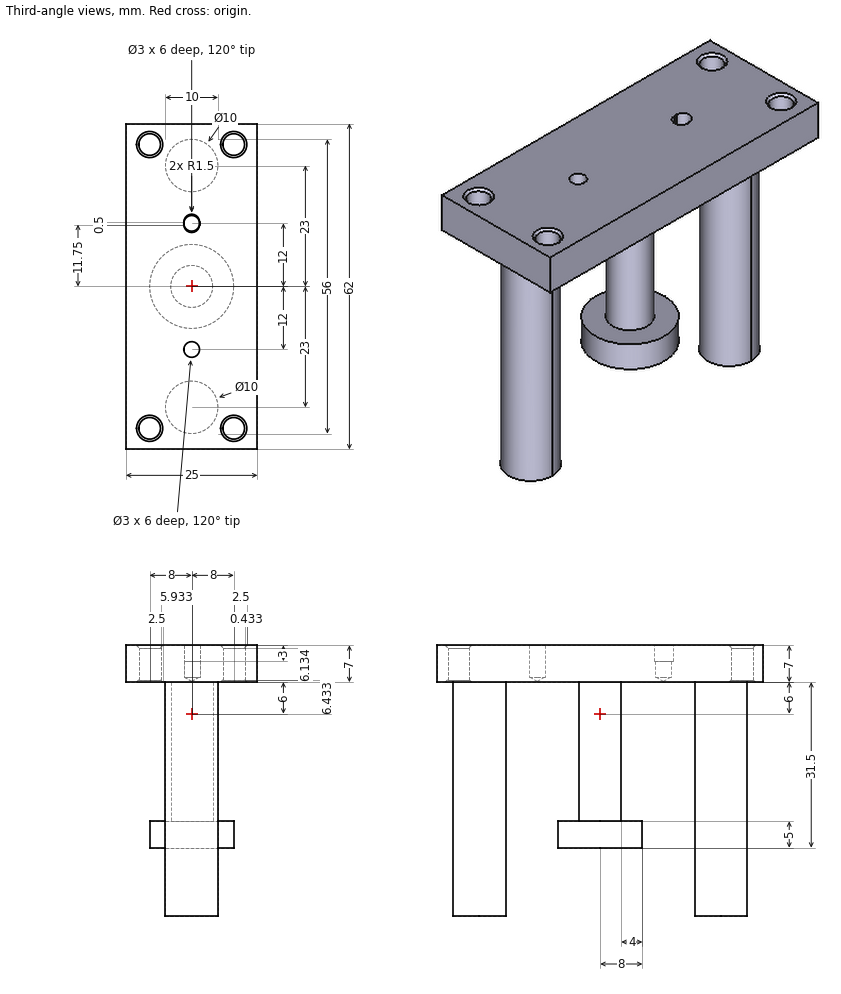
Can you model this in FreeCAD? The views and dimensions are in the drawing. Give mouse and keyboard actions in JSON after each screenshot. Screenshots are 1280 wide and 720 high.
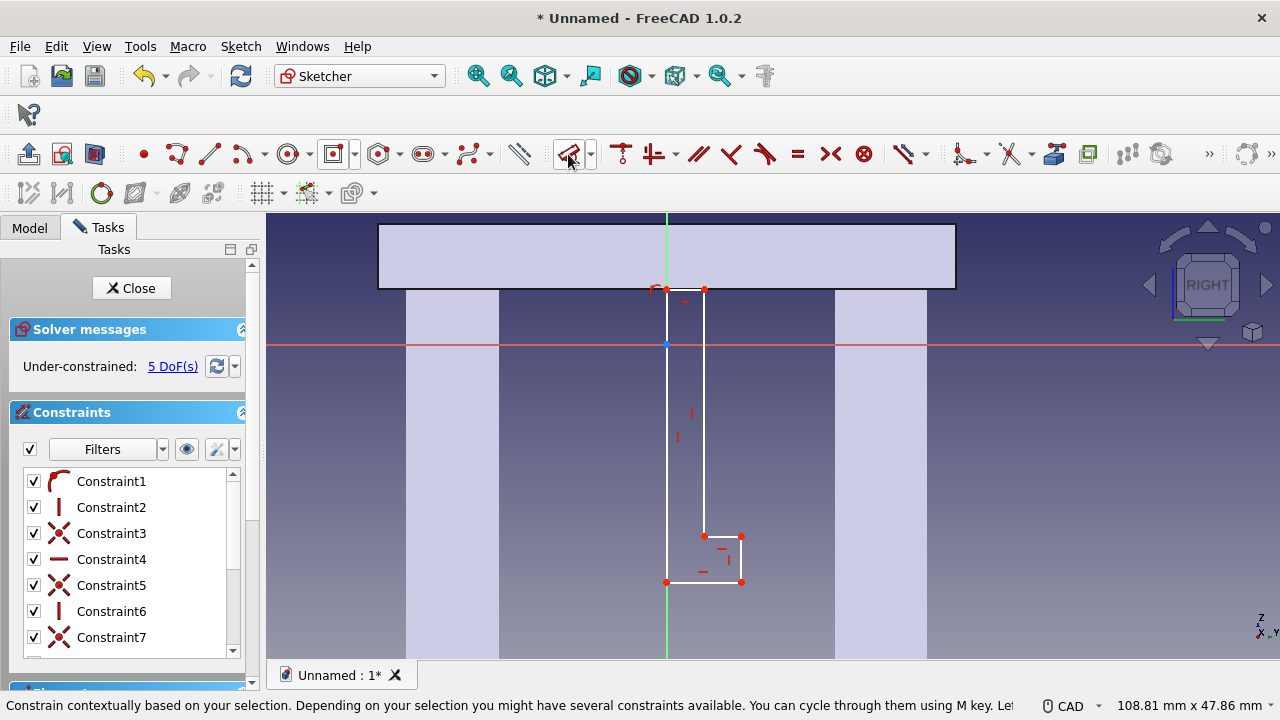
{"action": "left_click", "coordinate": [689, 583]}
{"action": "left_click", "coordinate": [704, 617]}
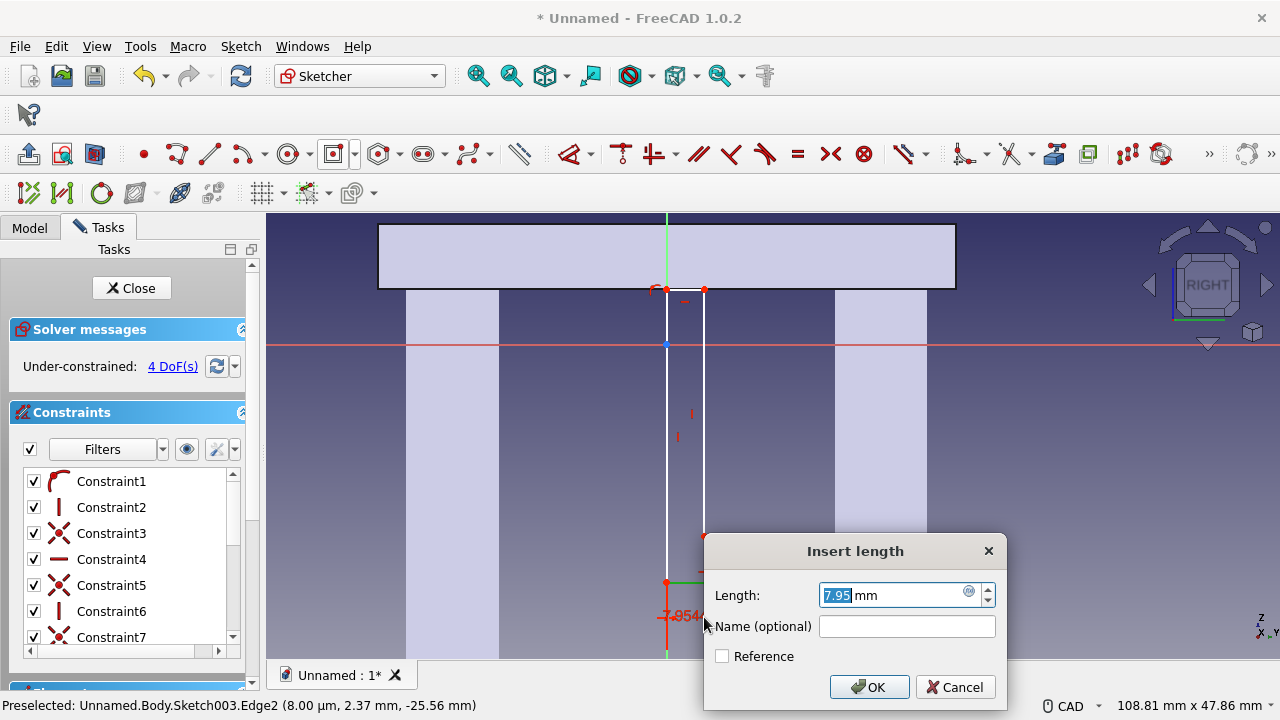
{"action": "type", "text": "8"}
{"action": "key", "text": "Return"}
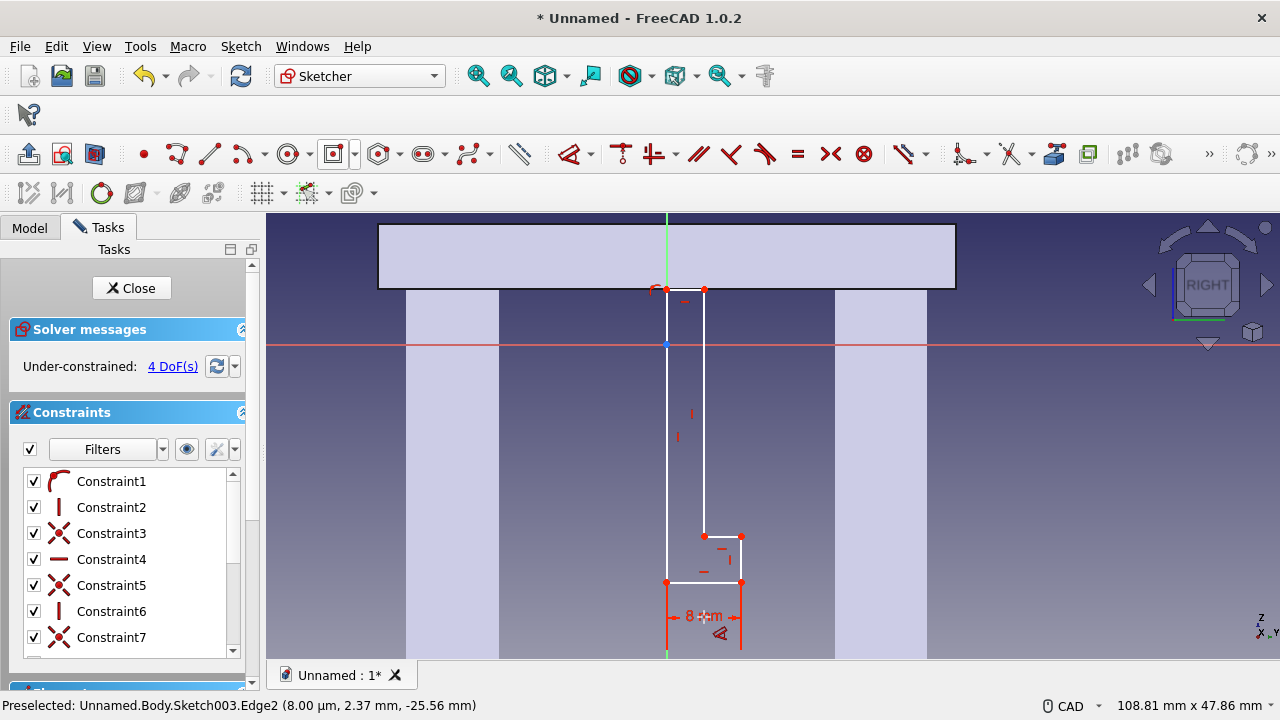
{"action": "left_click", "coordinate": [741, 569]}
{"action": "left_click", "coordinate": [775, 560]}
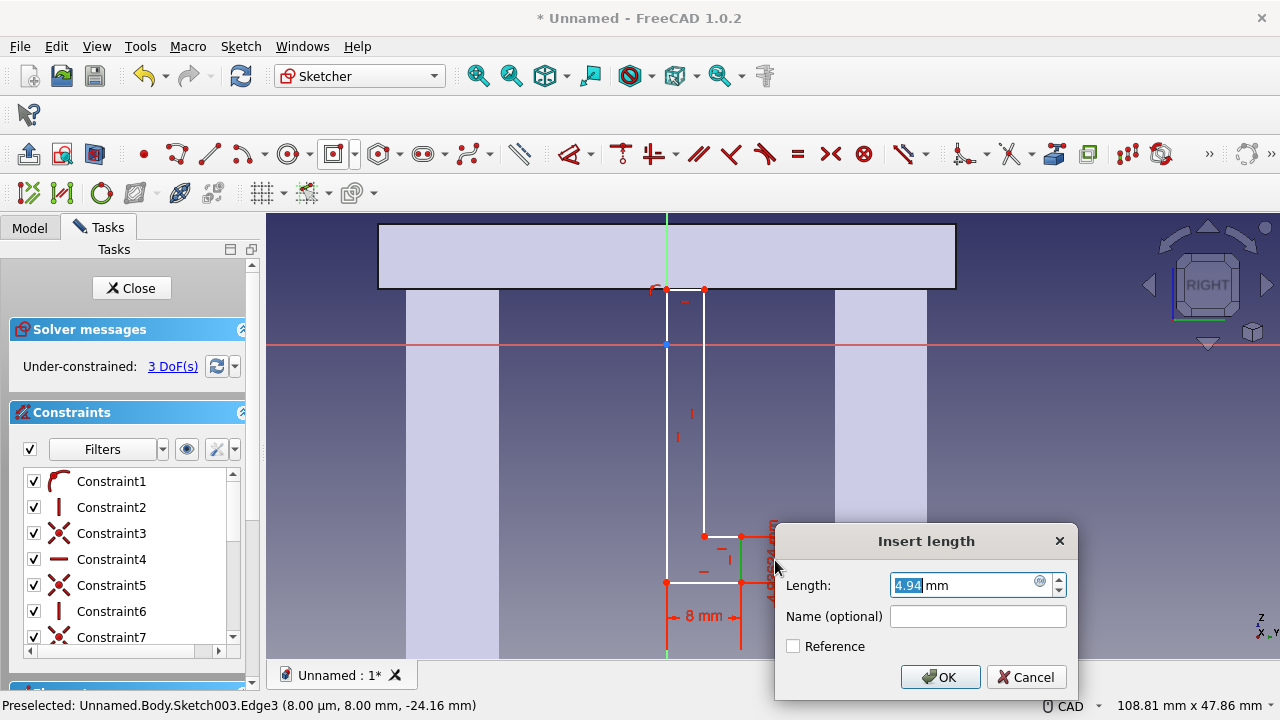
{"action": "type", "text": "5"}
{"action": "key", "text": "Return"}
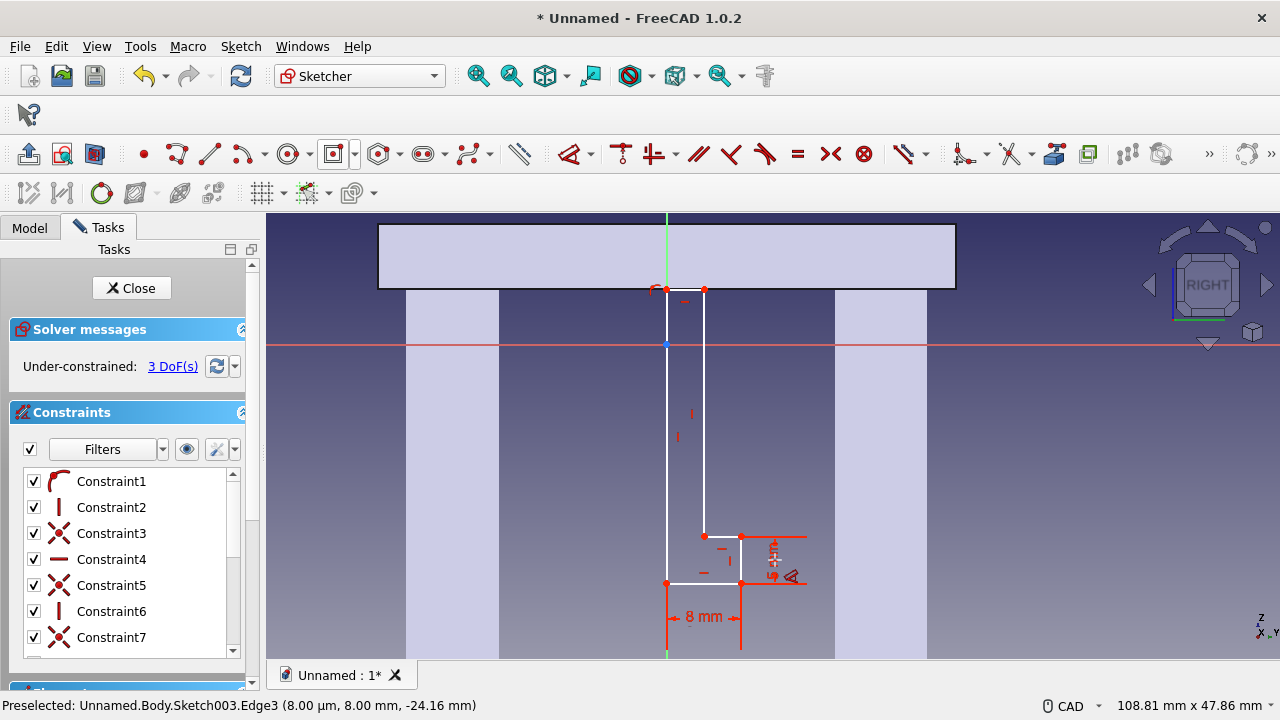
{"action": "scroll", "coordinate": [730, 537], "scroll_direction": "up", "scroll_amount": 2}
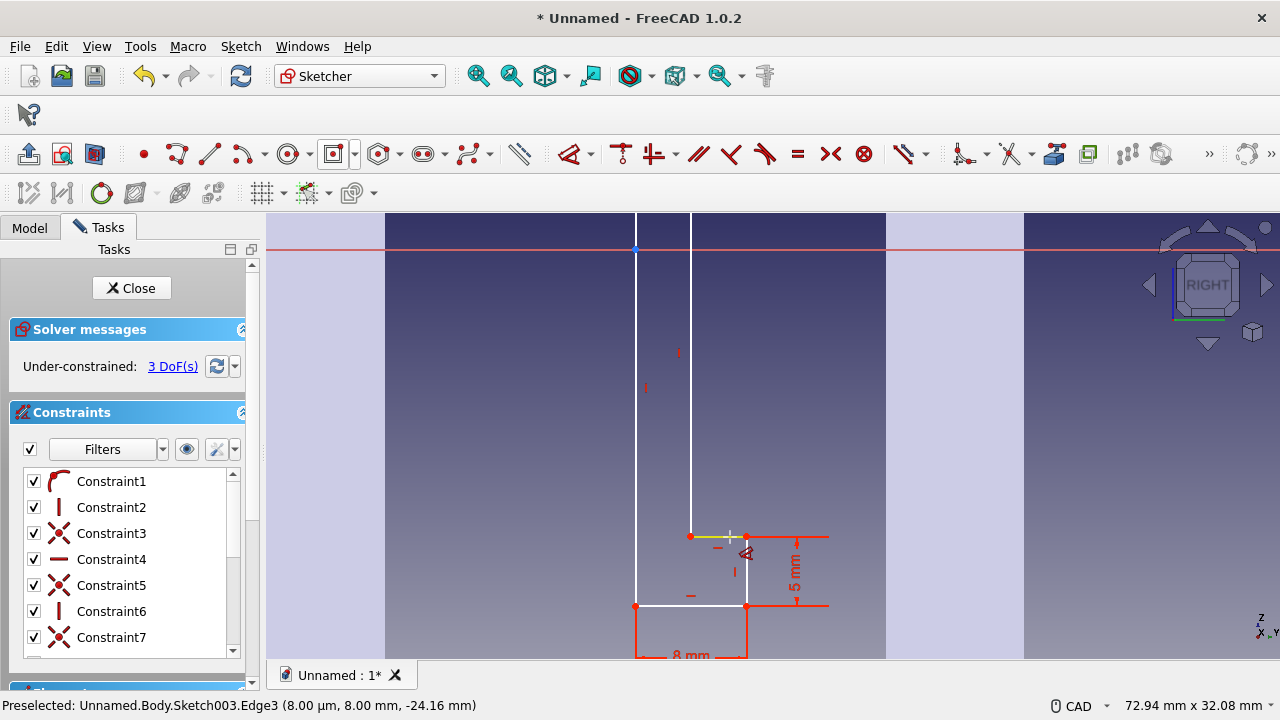
{"action": "left_click", "coordinate": [730, 537]}
{"action": "left_click", "coordinate": [719, 571]}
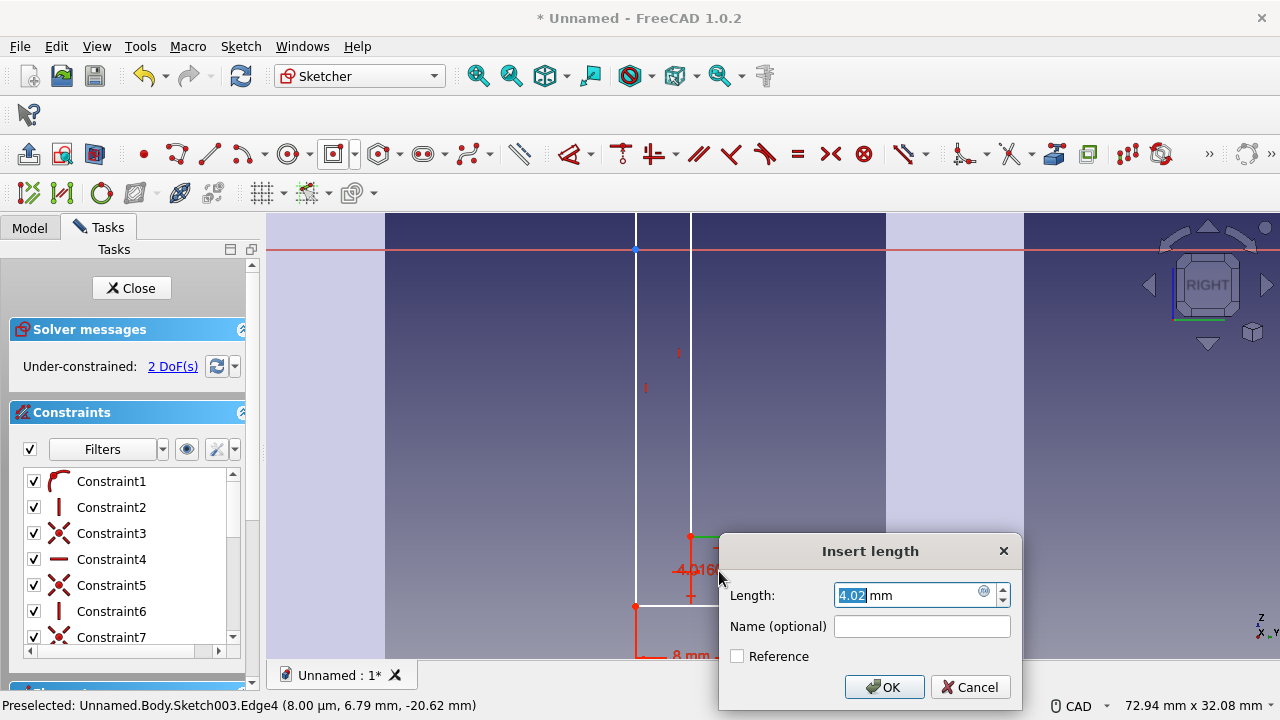
{"action": "type", "text": "4"}
{"action": "key", "text": "Return"}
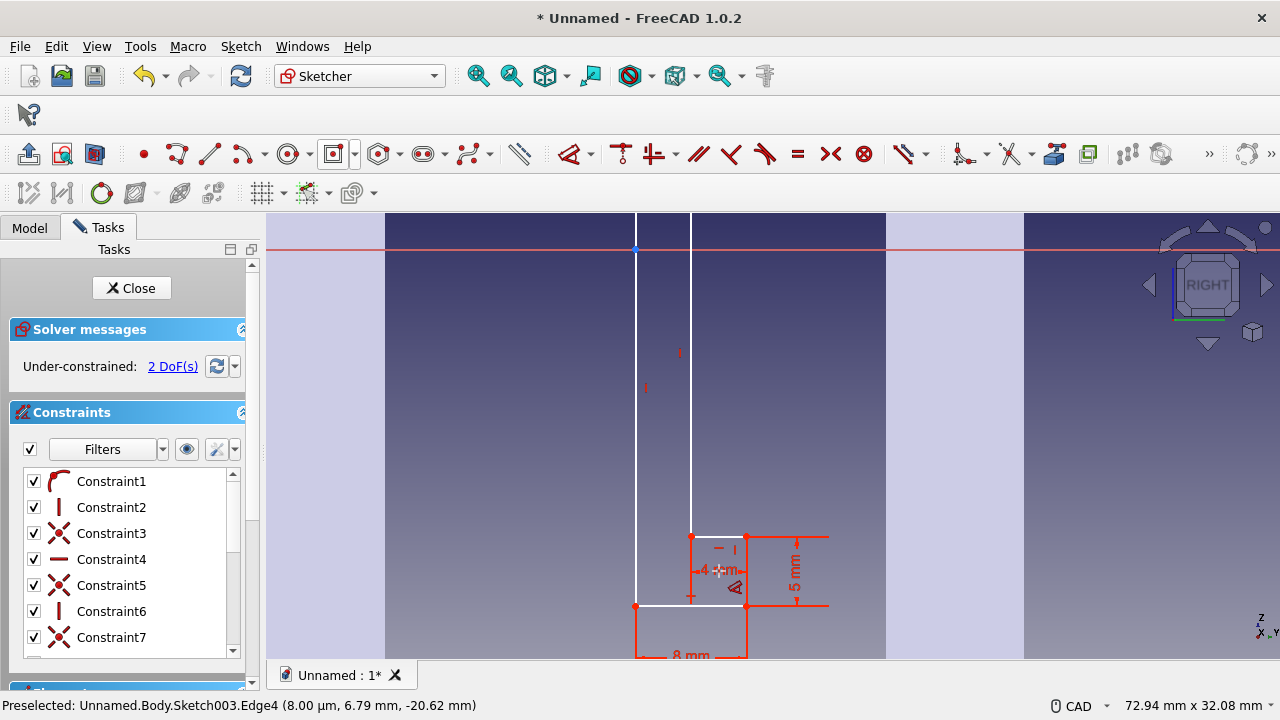
{"action": "scroll", "coordinate": [732, 539], "scroll_direction": "down", "scroll_amount": 2}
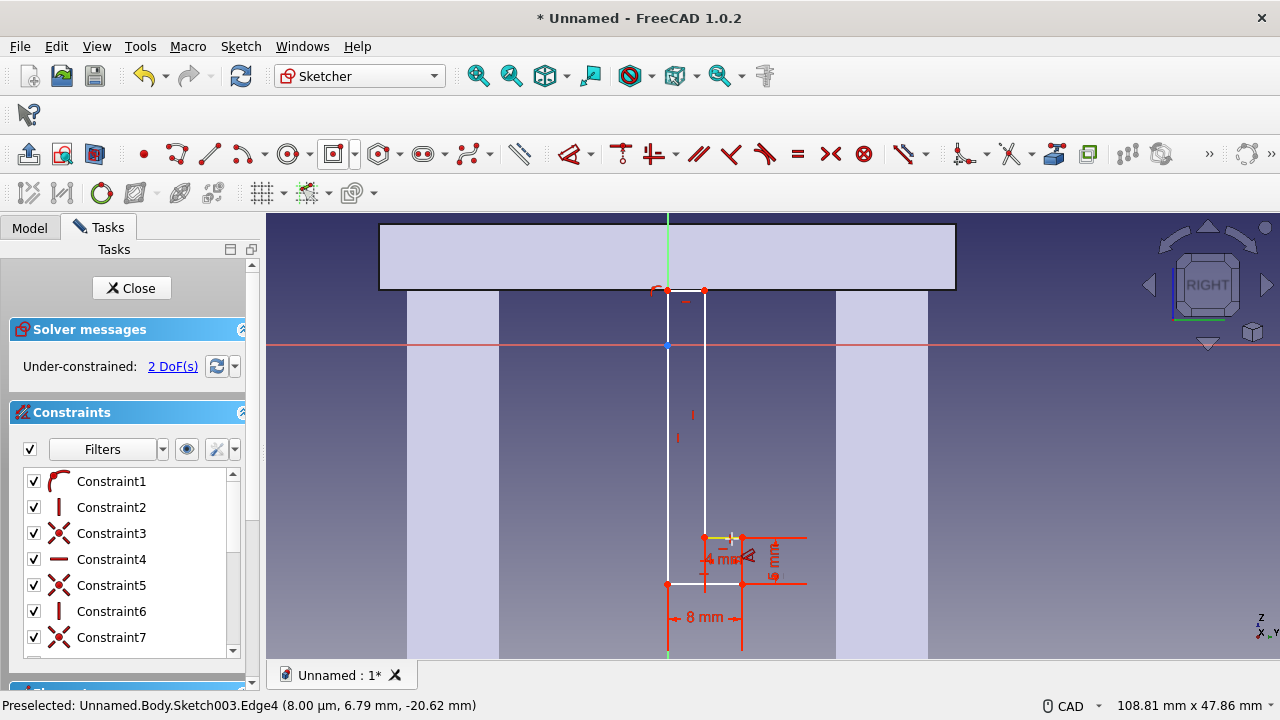
{"action": "left_click", "coordinate": [668, 291]}
{"action": "left_click", "coordinate": [634, 318]}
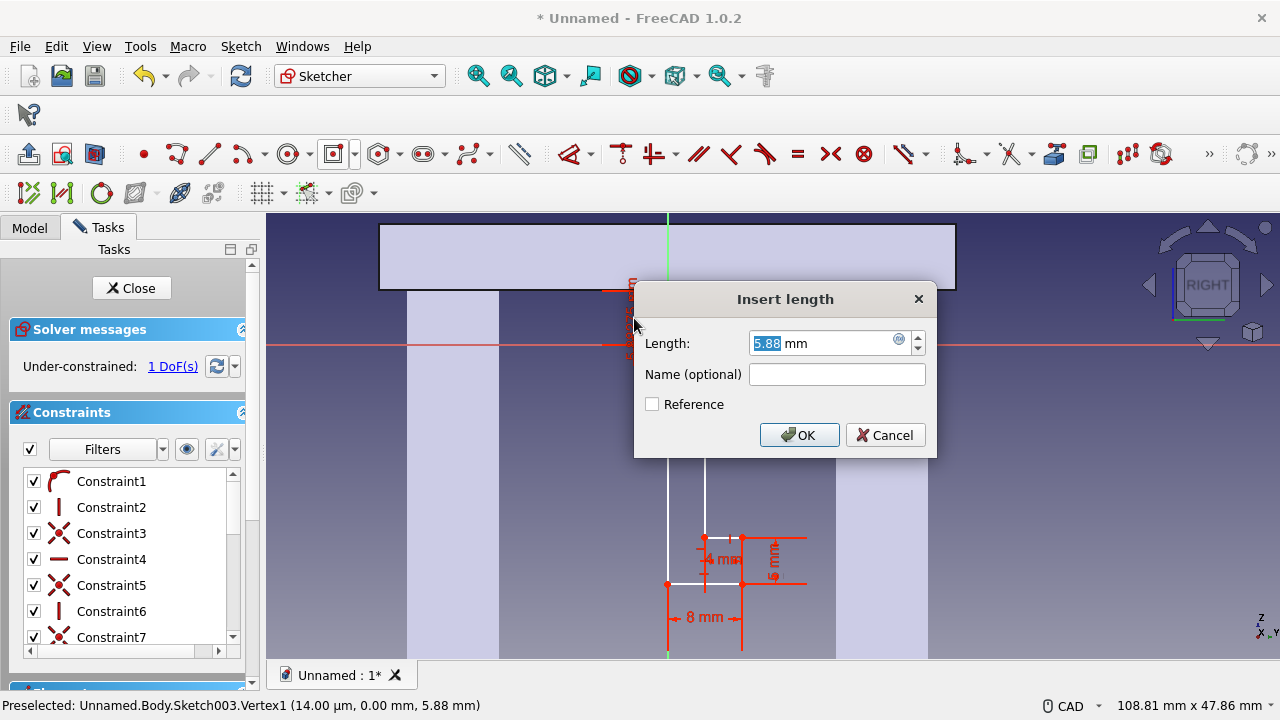
{"action": "type", "text": "6"}
{"action": "key", "text": "Return"}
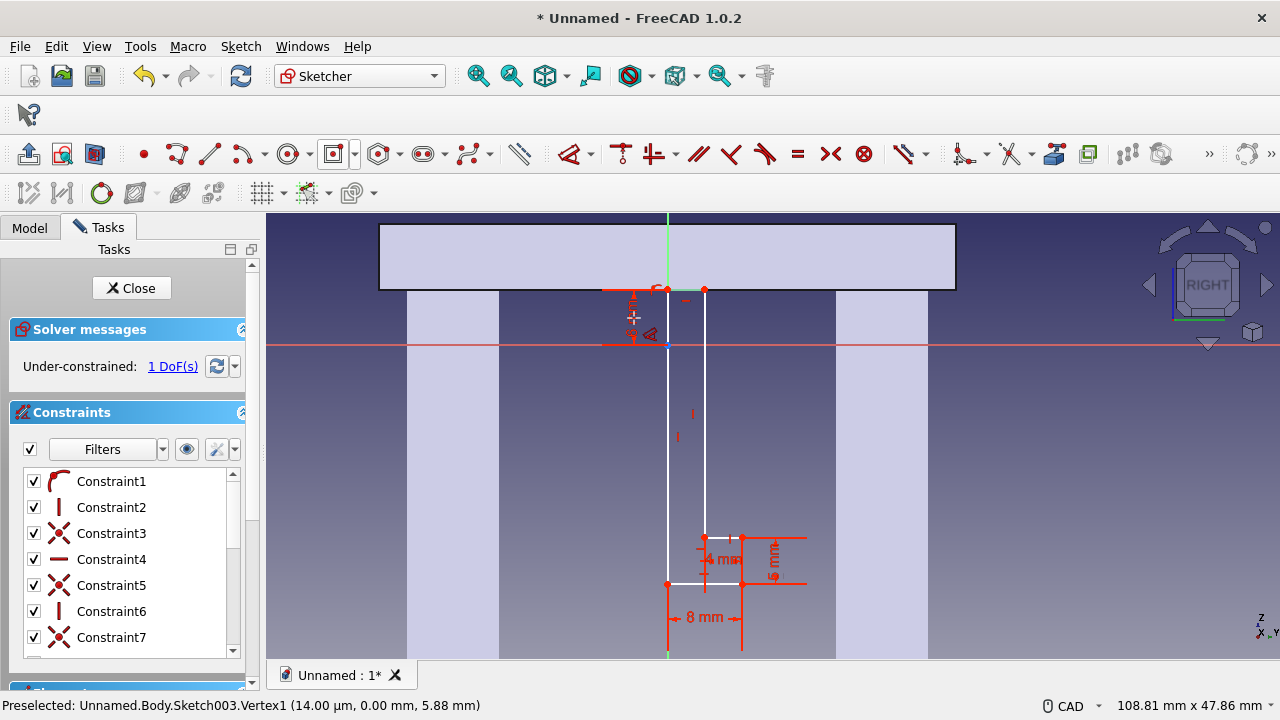
{"action": "left_click", "coordinate": [668, 378]}
{"action": "left_click", "coordinate": [634, 437]}